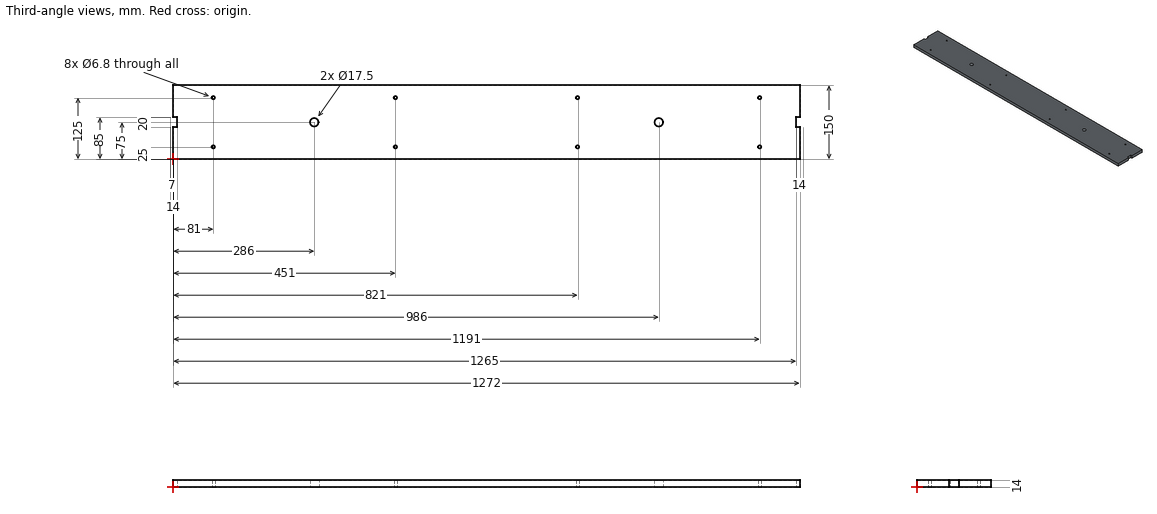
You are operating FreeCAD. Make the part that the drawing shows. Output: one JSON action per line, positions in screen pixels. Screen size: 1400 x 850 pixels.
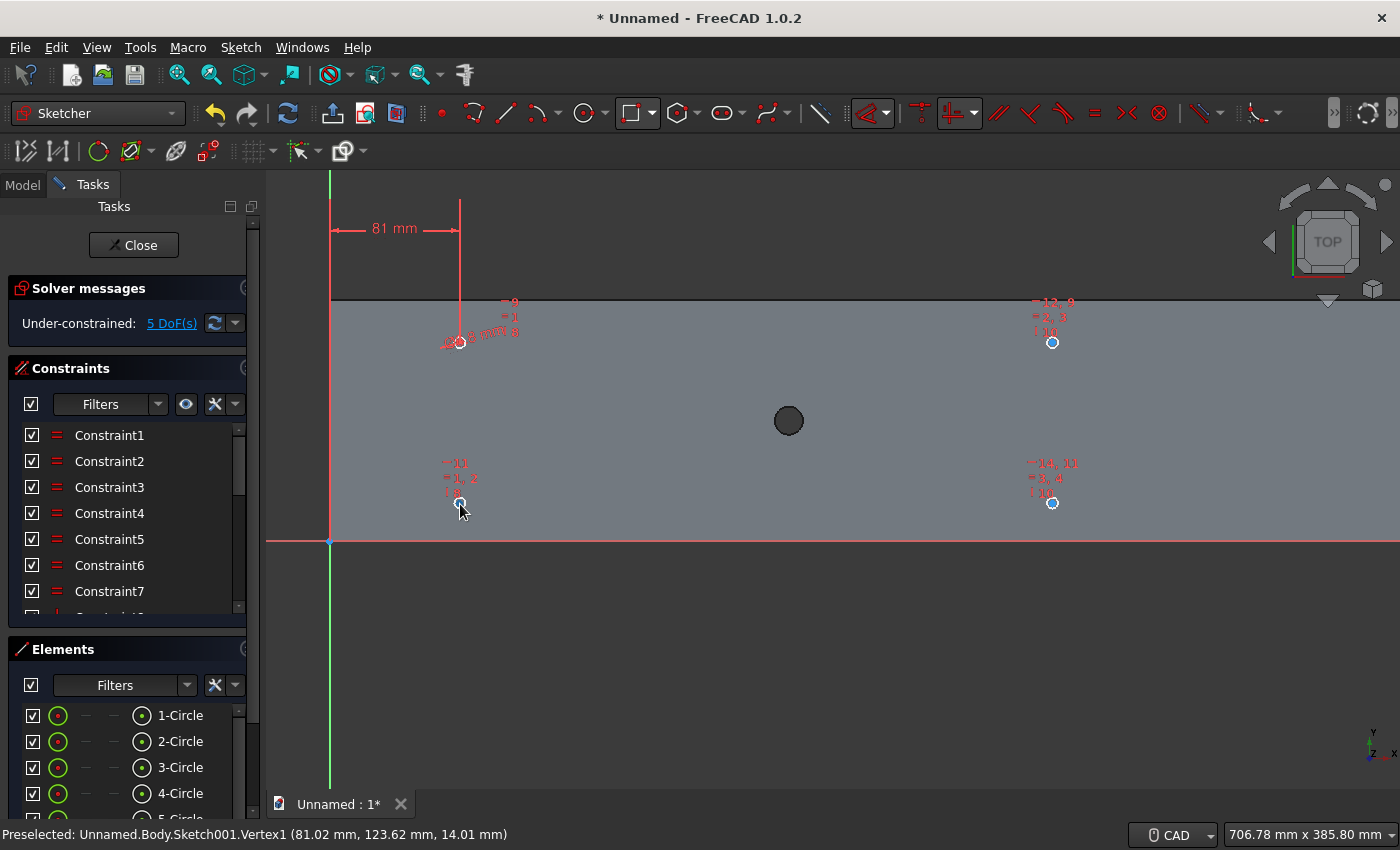
{"action": "left_click", "coordinate": [460, 503]}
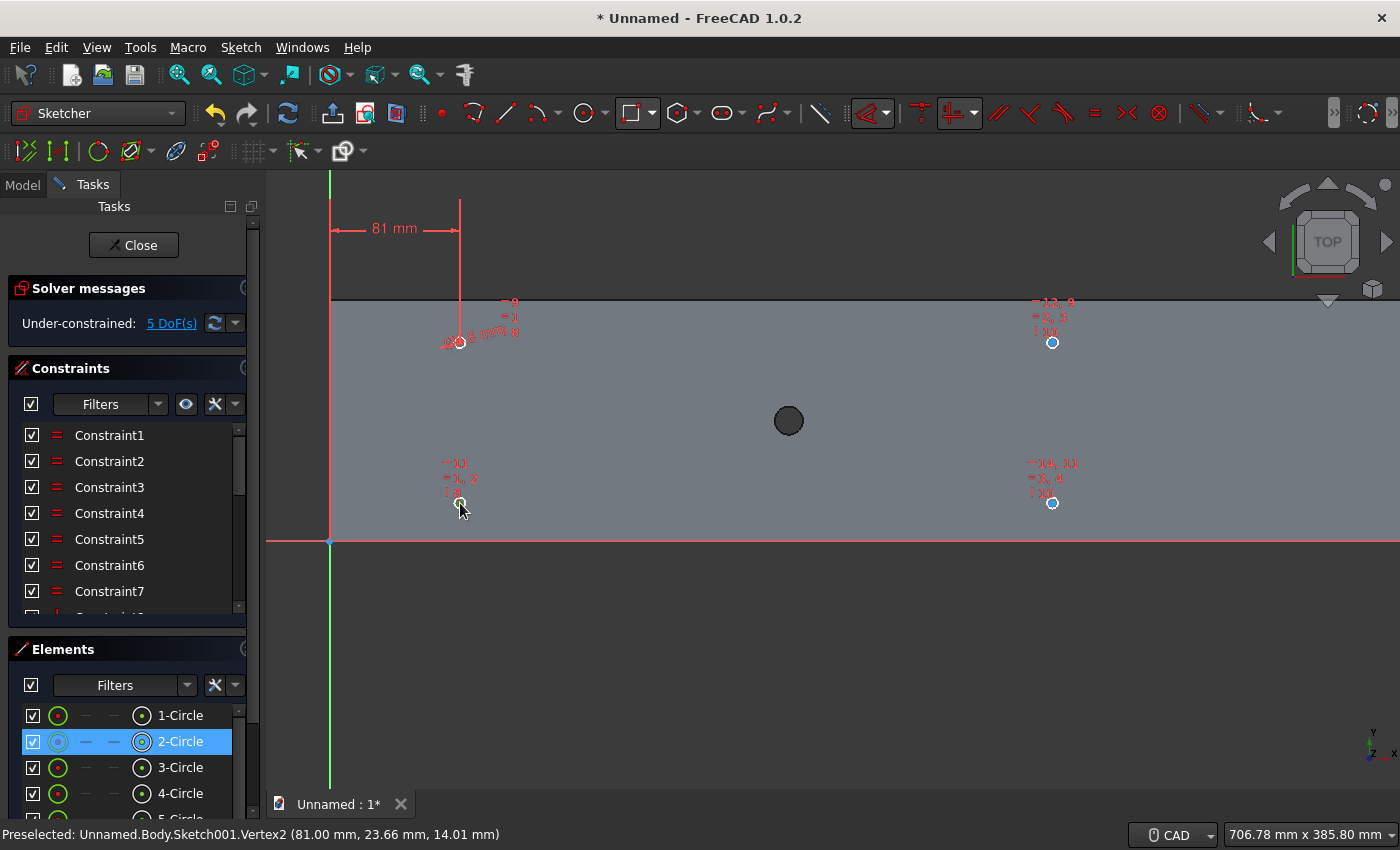
{"action": "key", "text": "i"}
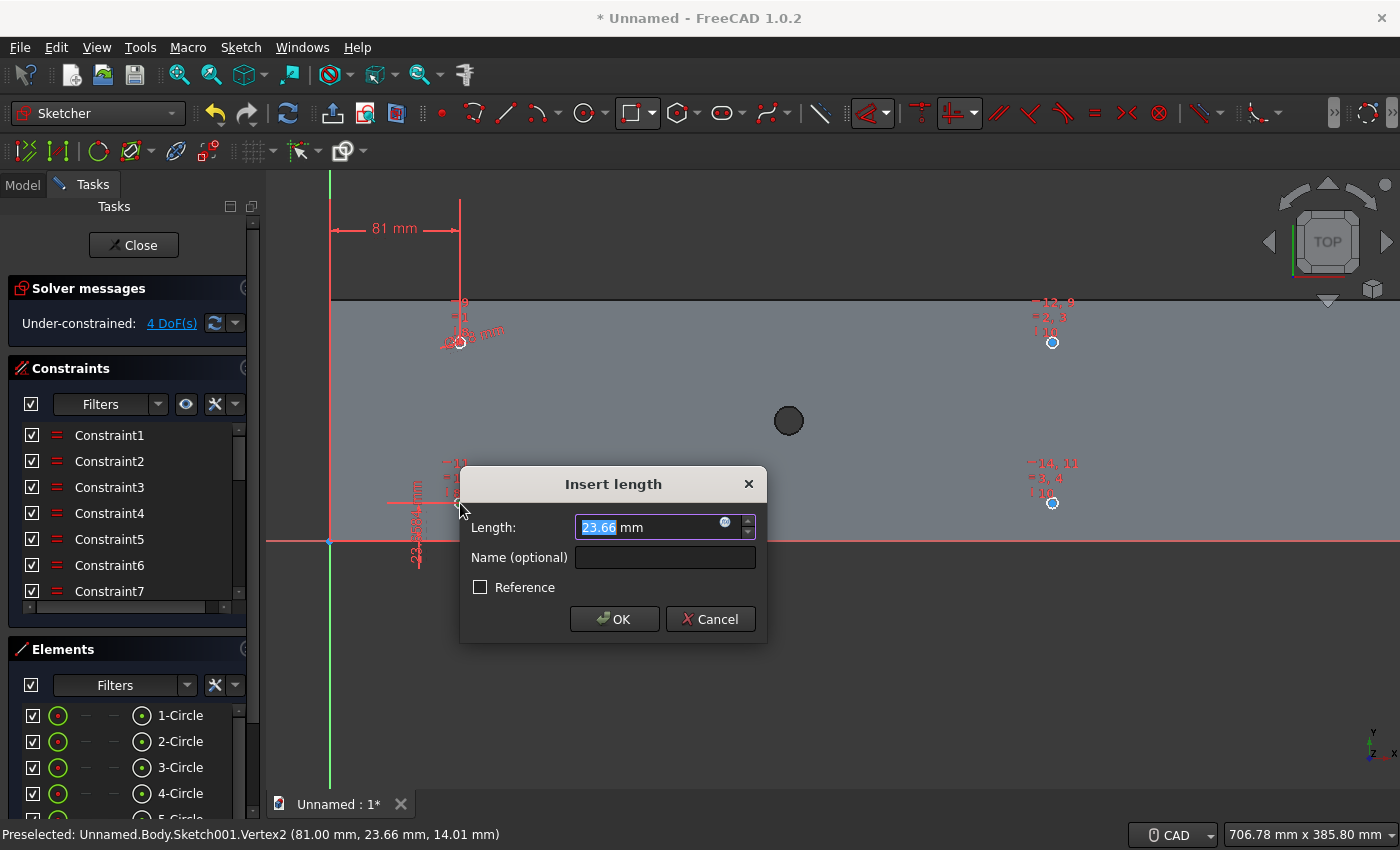
{"action": "type", "text": "25"}
{"action": "key", "text": "Return"}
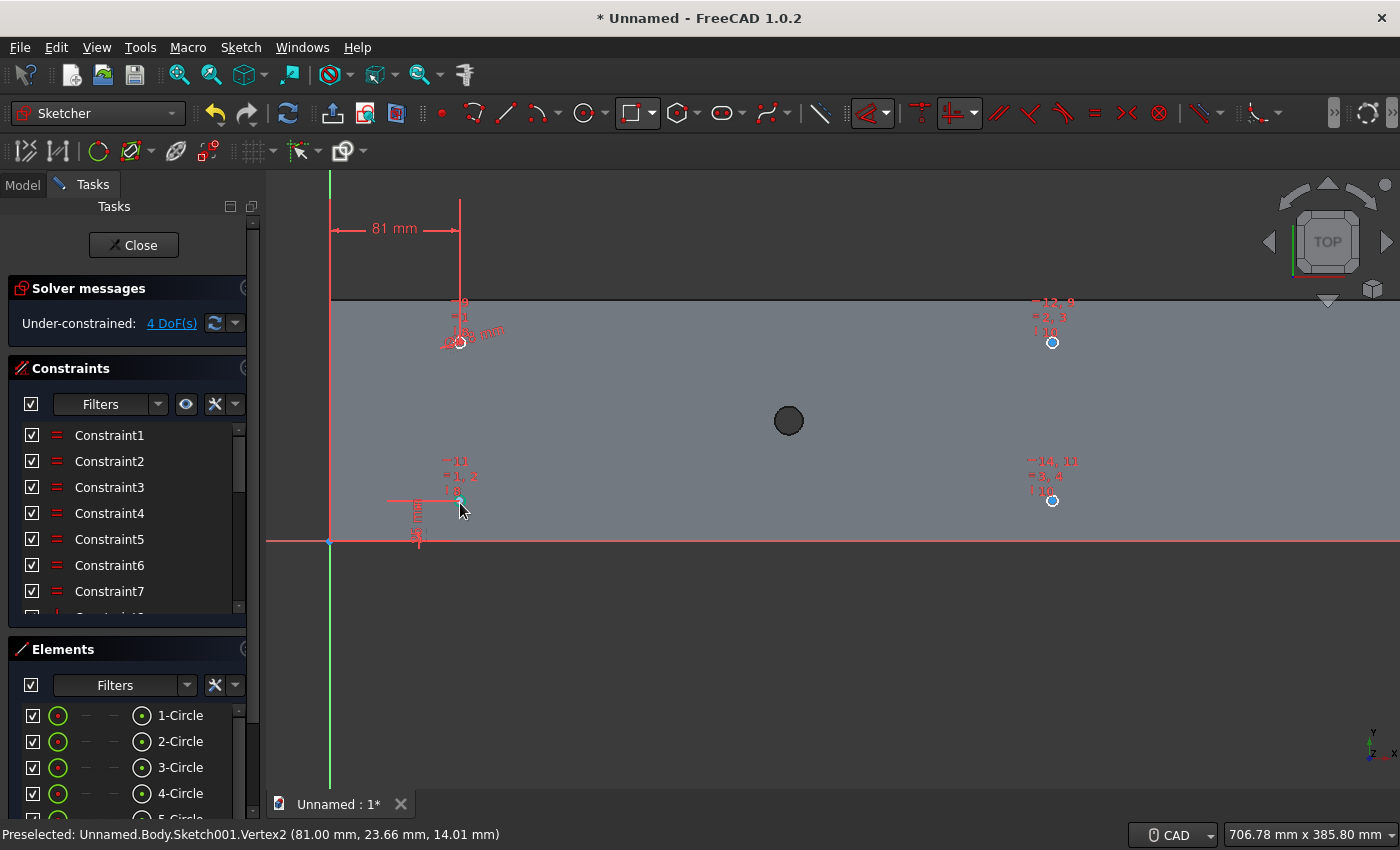
{"action": "left_click", "coordinate": [460, 343]}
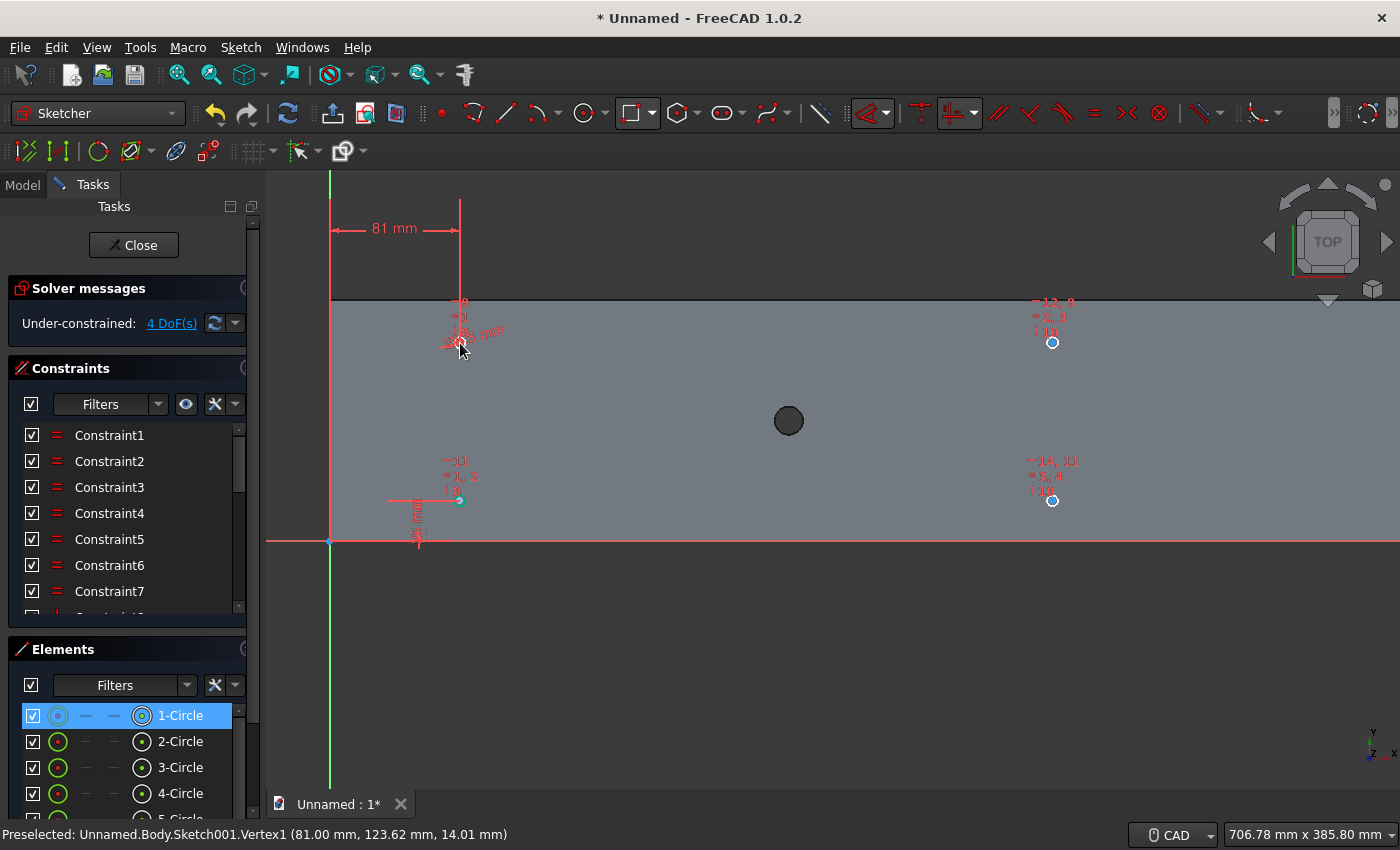
{"action": "key", "text": "i"}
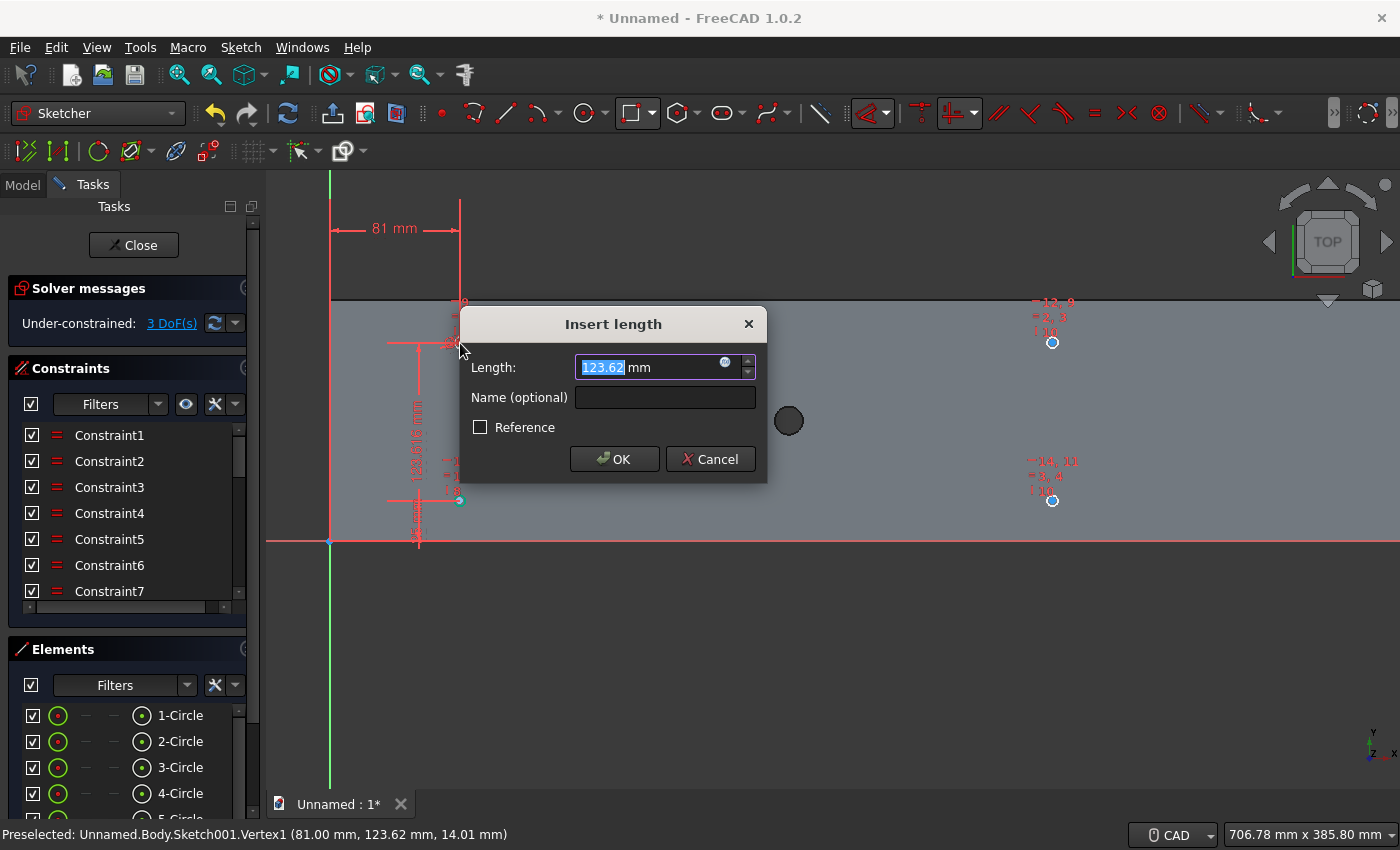
{"action": "type", "text": "125"}
{"action": "key", "text": "Return"}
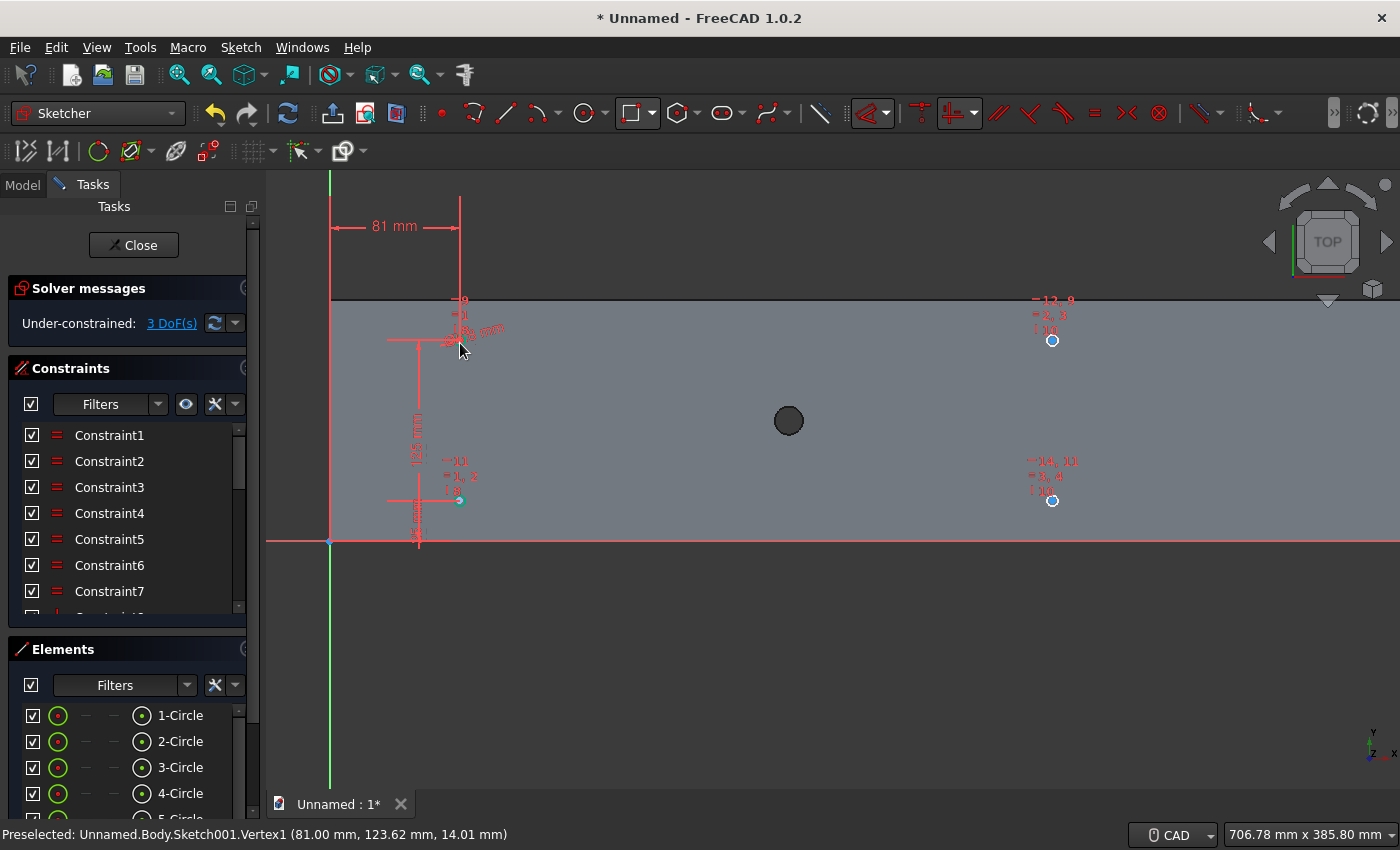
{"action": "left_click", "coordinate": [1053, 340]}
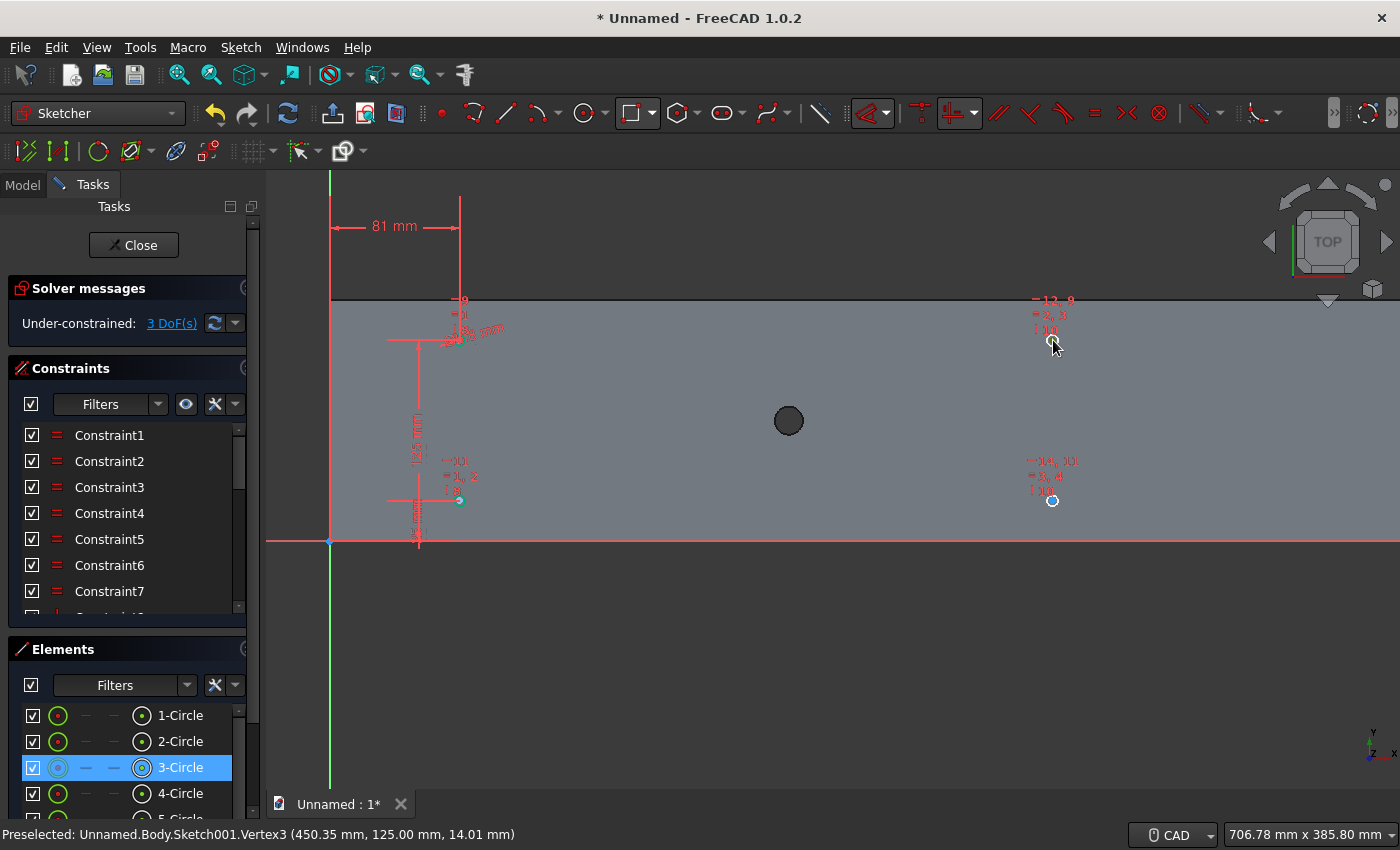
{"action": "left_click", "coordinate": [888, 114]}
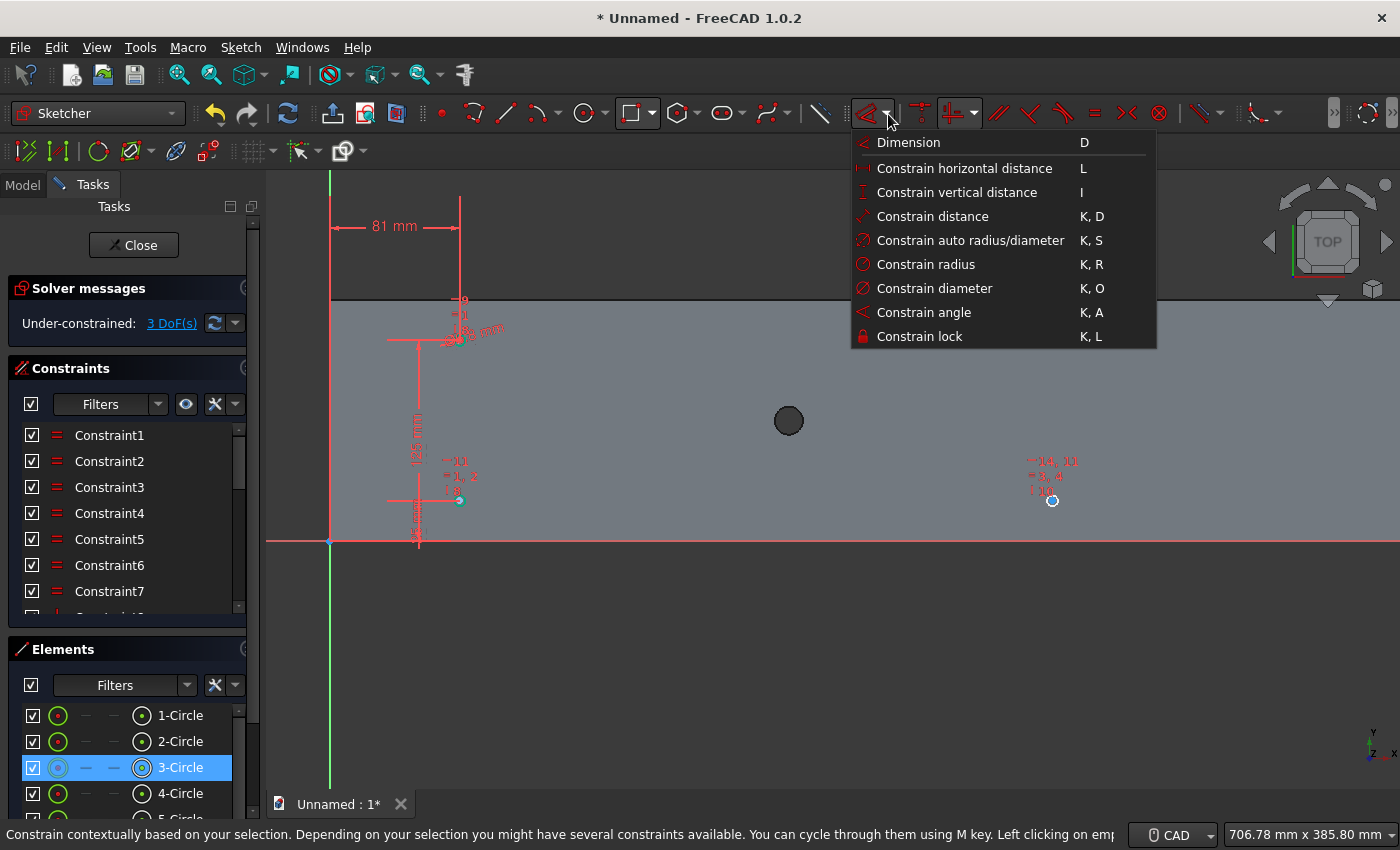
{"action": "left_click", "coordinate": [1004, 168]}